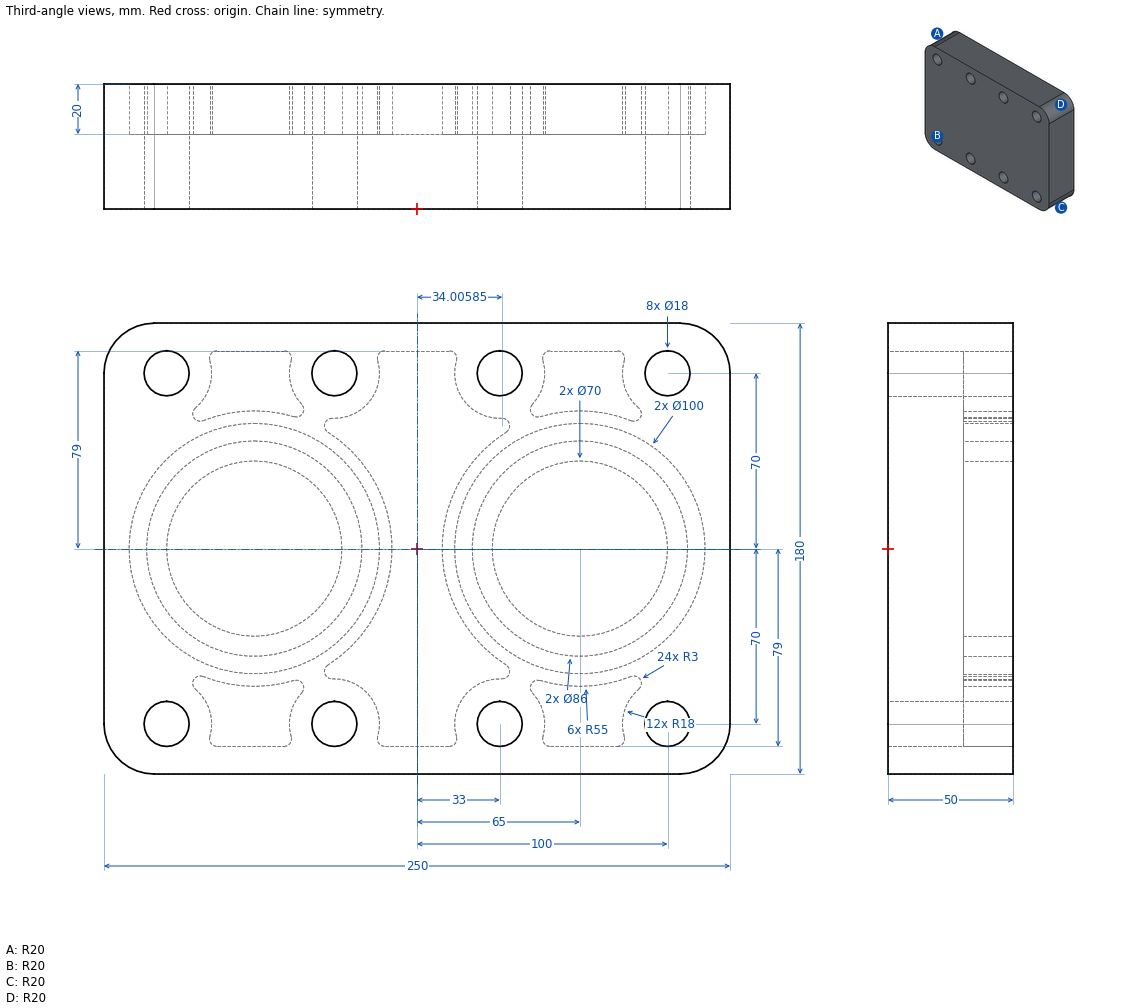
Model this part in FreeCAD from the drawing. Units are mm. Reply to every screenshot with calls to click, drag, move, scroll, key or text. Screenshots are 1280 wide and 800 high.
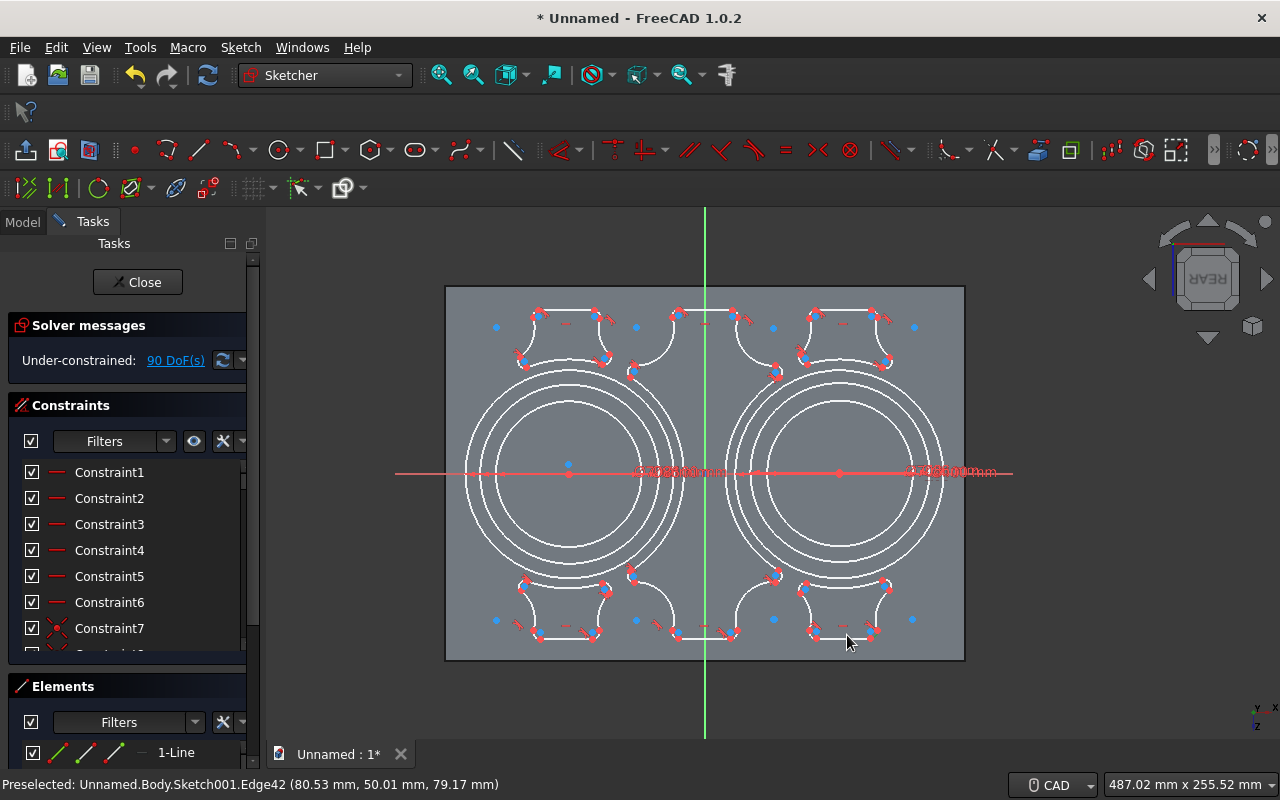
click(881, 601)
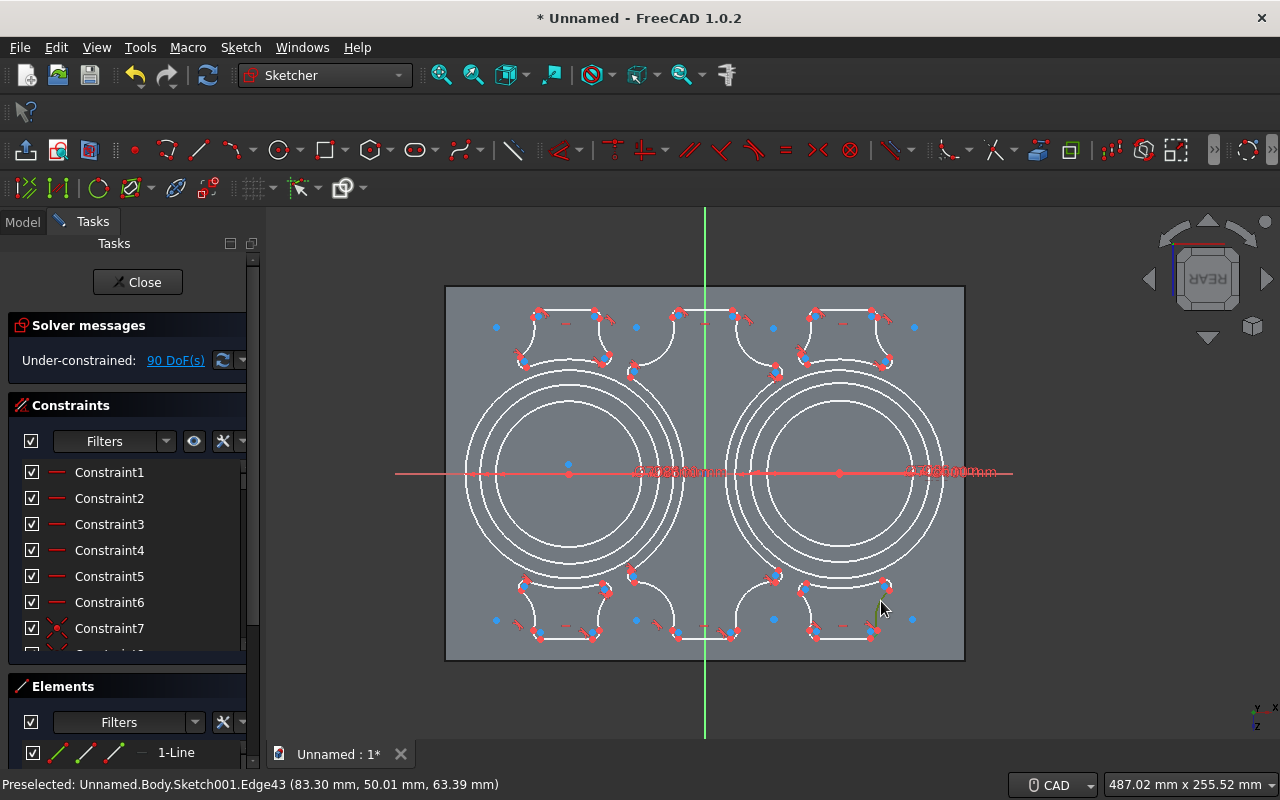
click(754, 150)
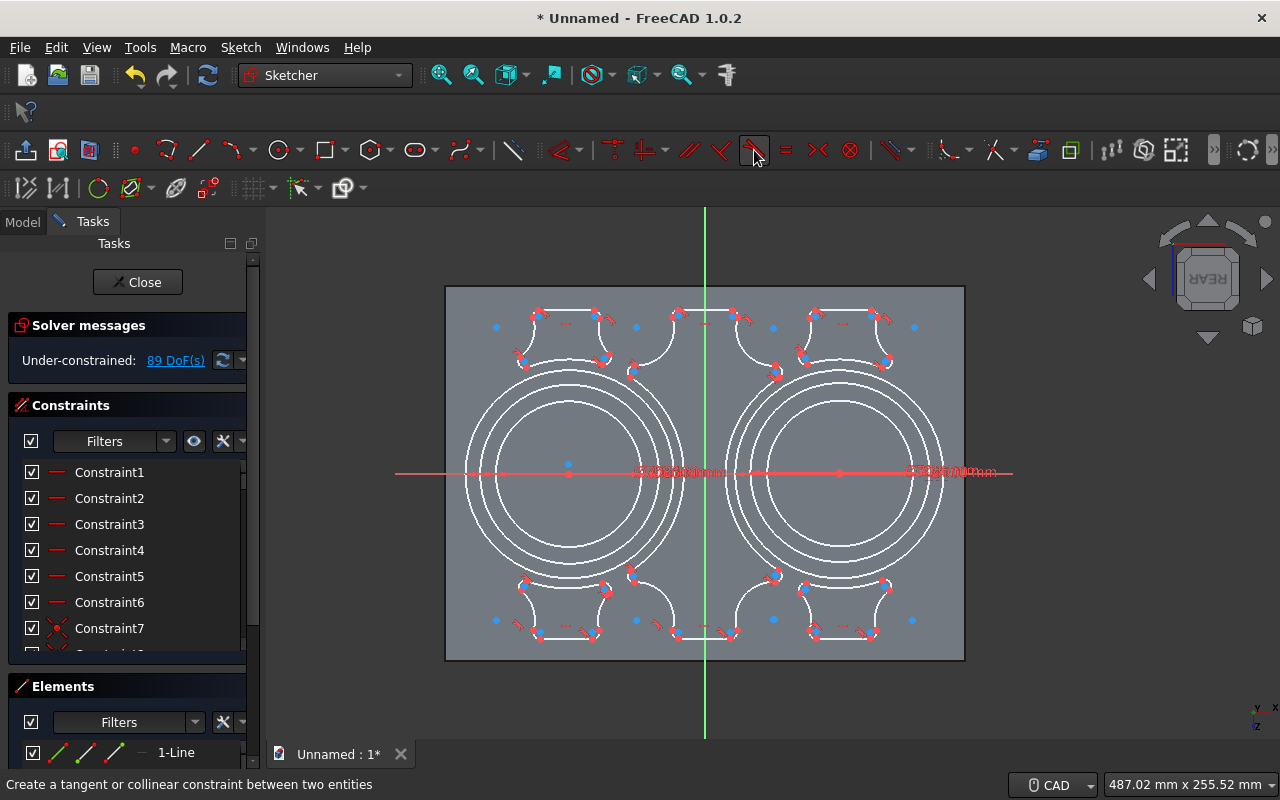
click(880, 601)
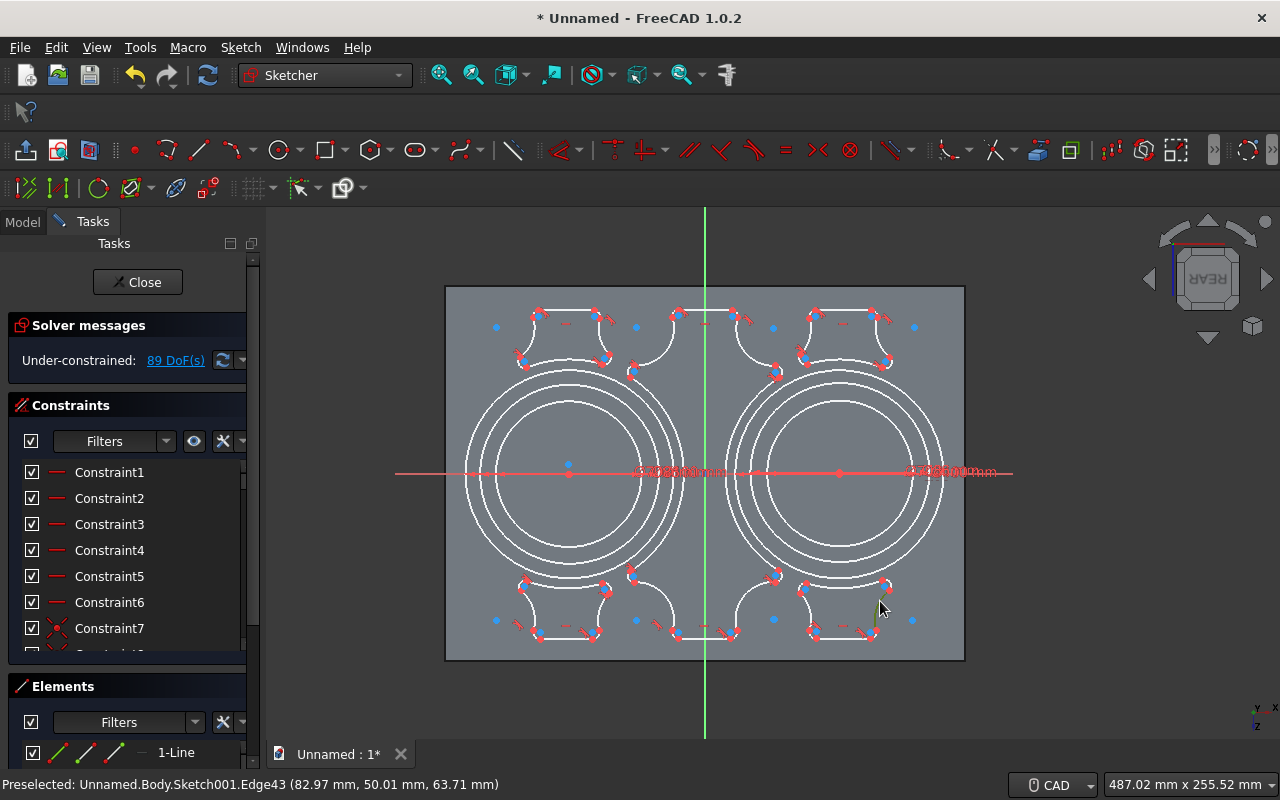
scroll(890, 583, up, 4)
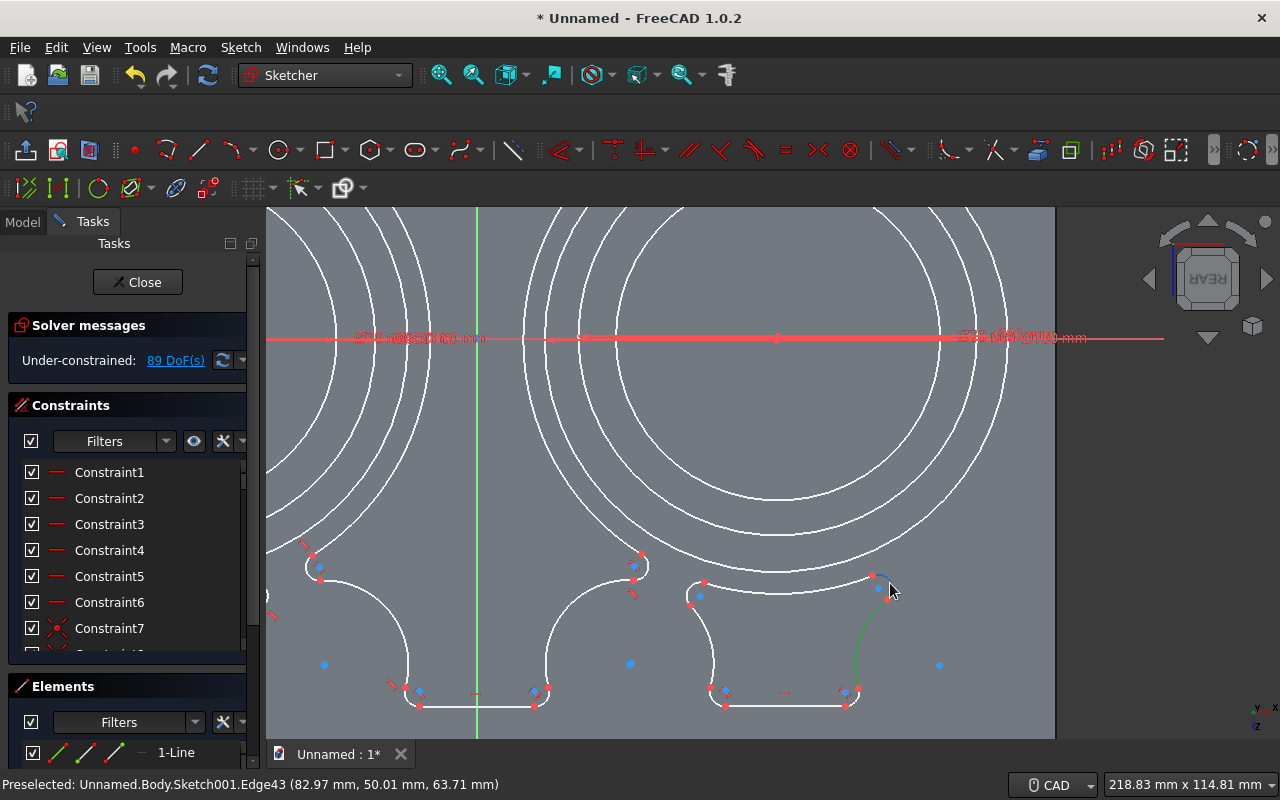
click(890, 581)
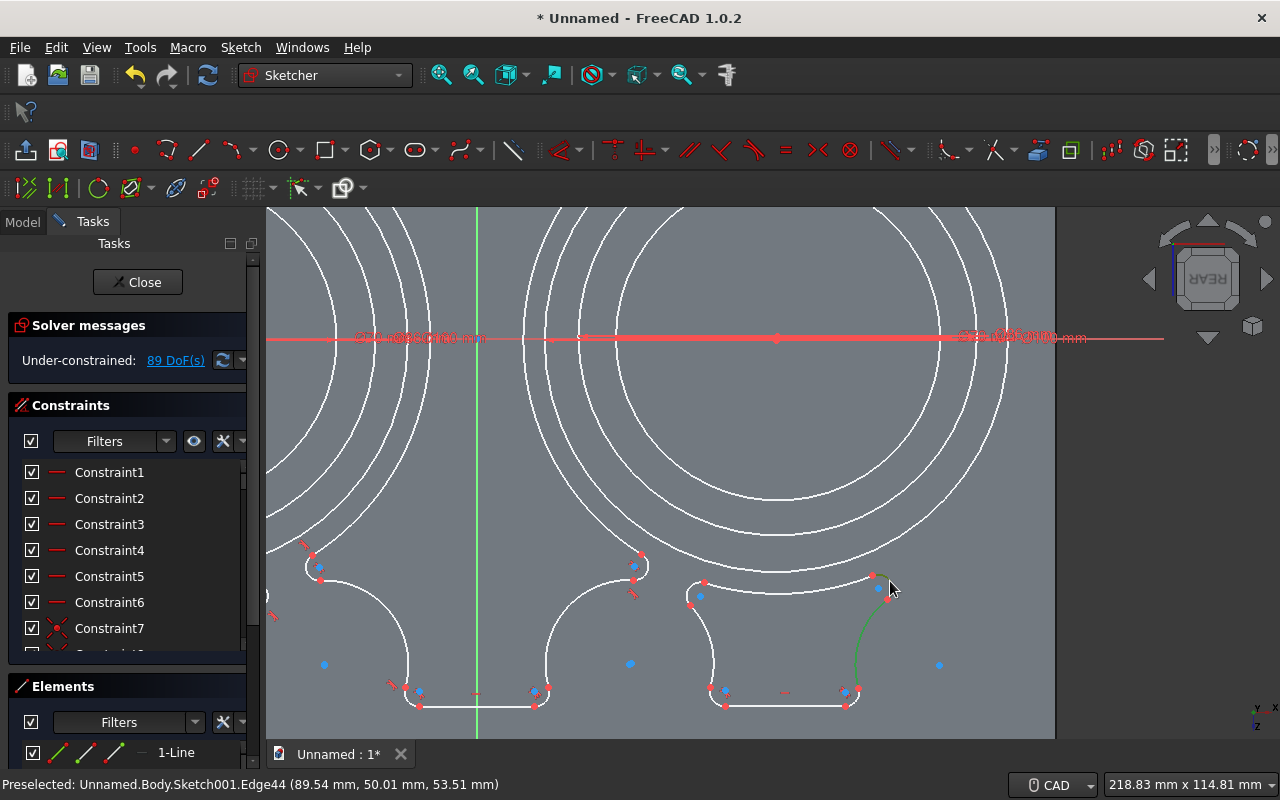
click(754, 150)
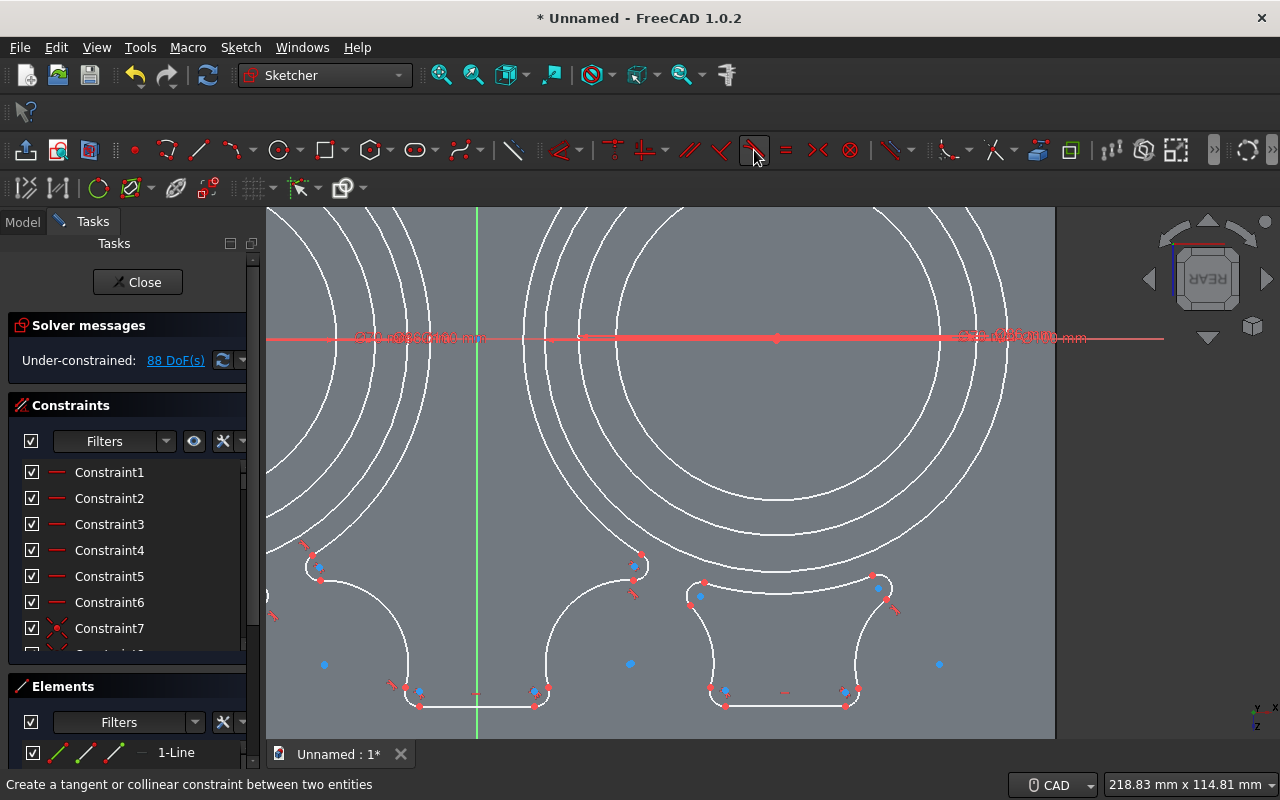
click(892, 589)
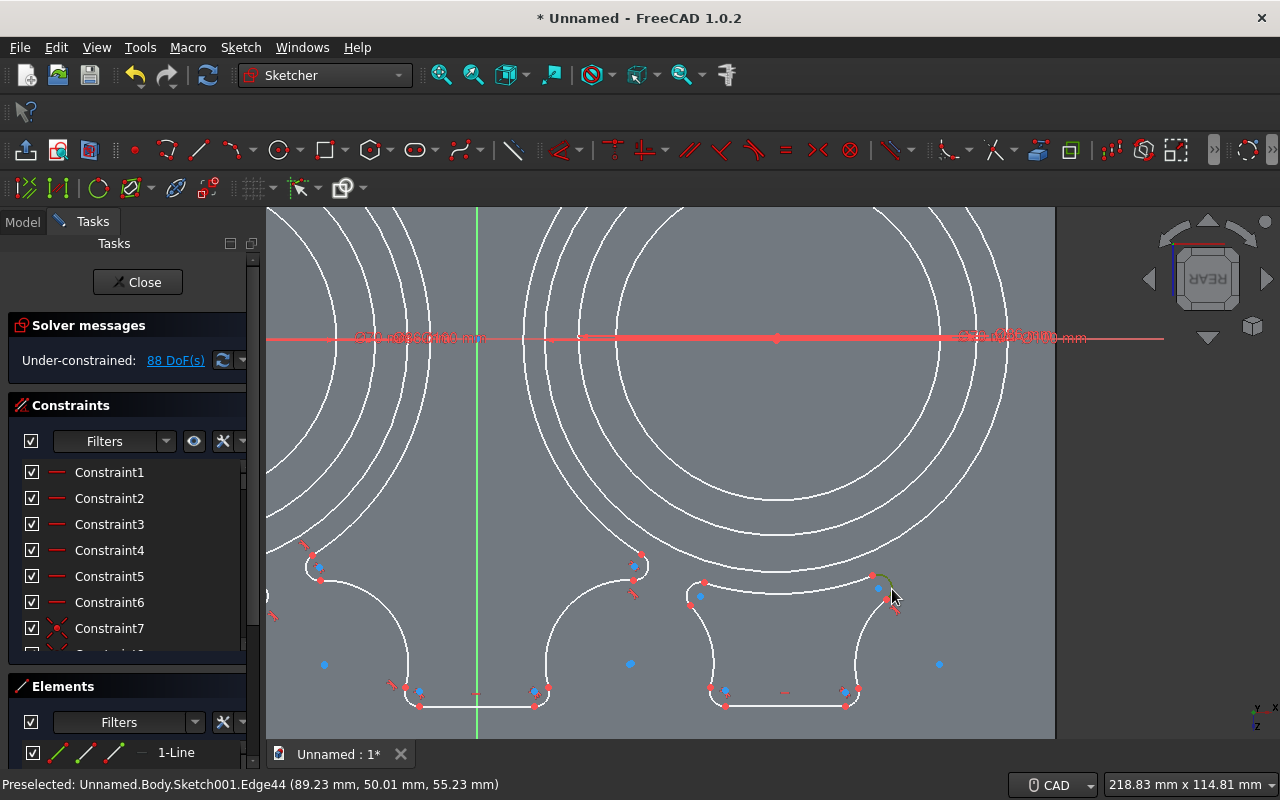
click(755, 593)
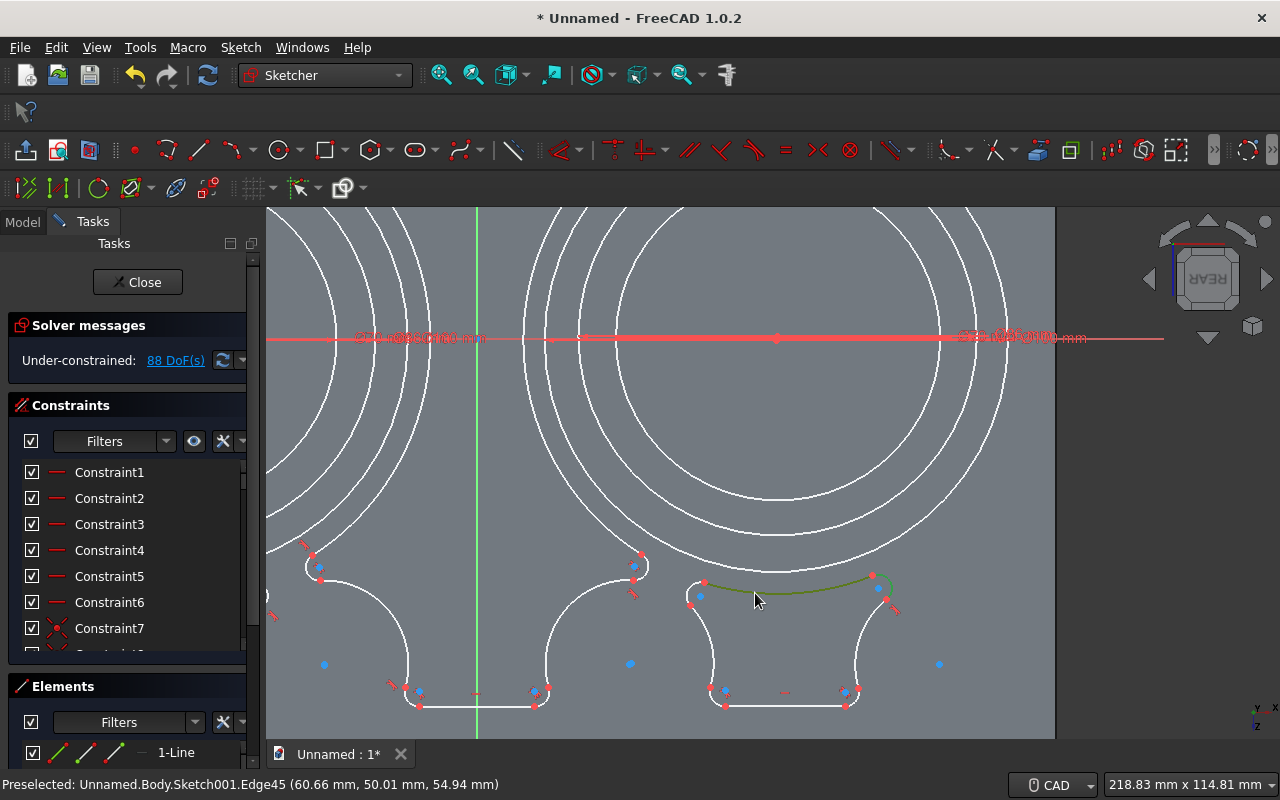
click(754, 150)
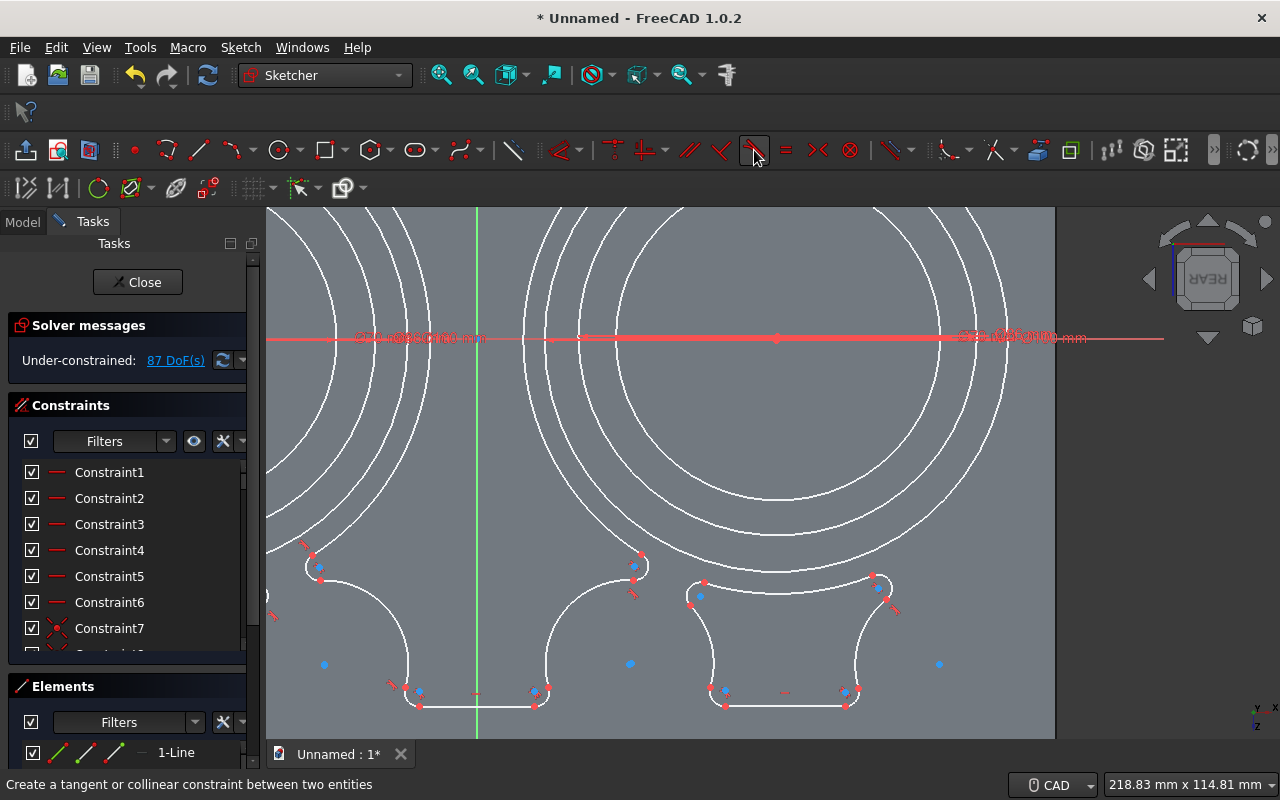
click(755, 593)